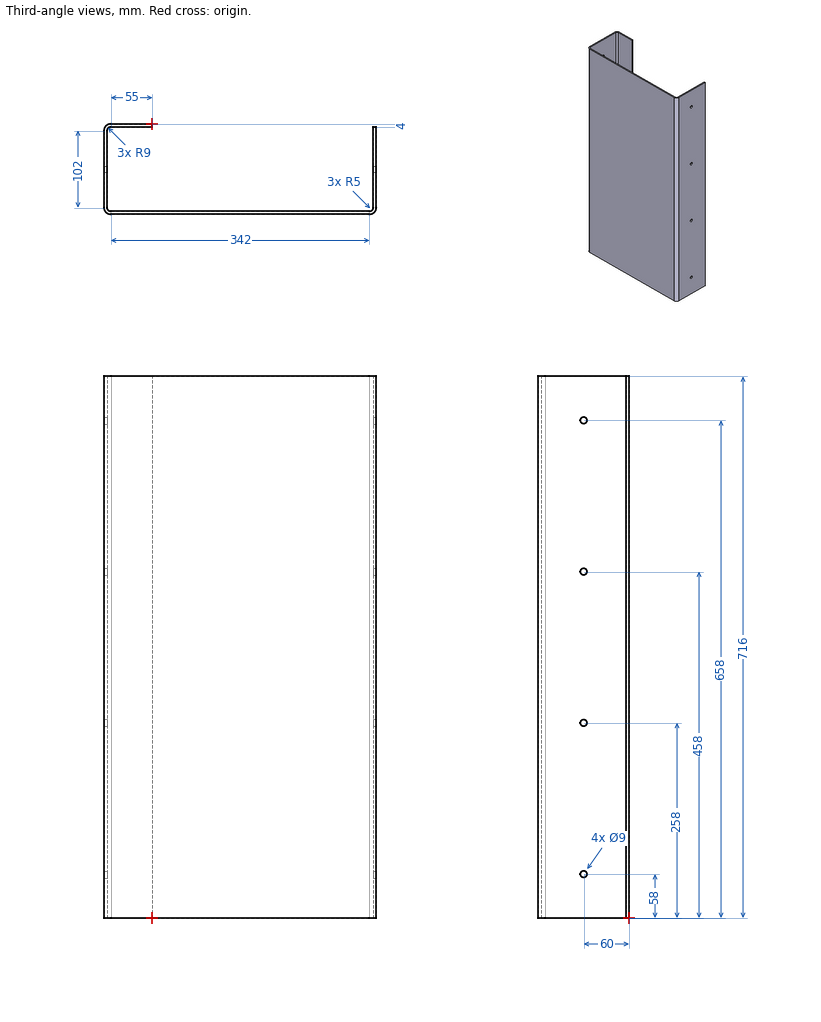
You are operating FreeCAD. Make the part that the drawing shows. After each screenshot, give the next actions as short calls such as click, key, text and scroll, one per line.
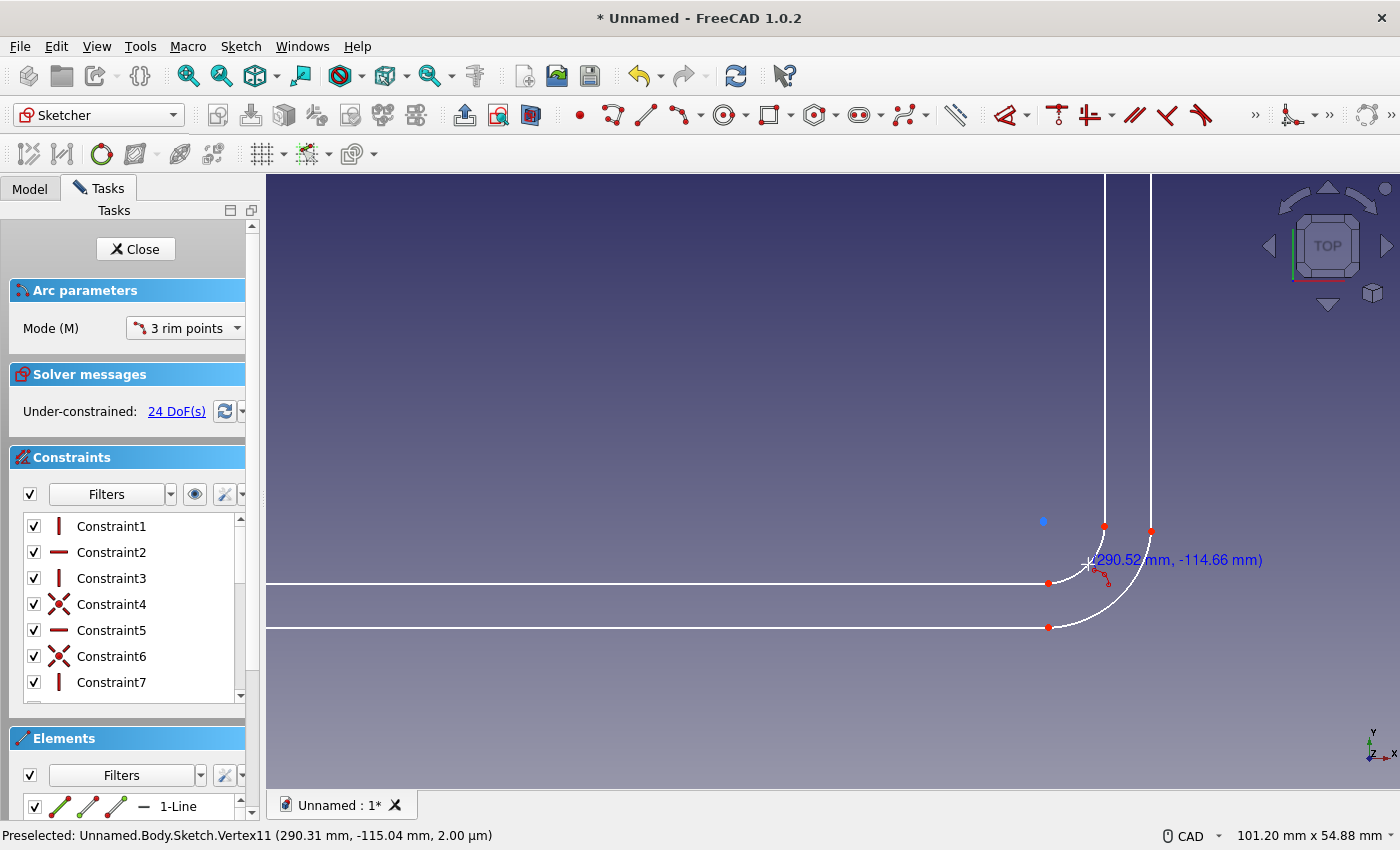
scroll(1088, 586, down, 9)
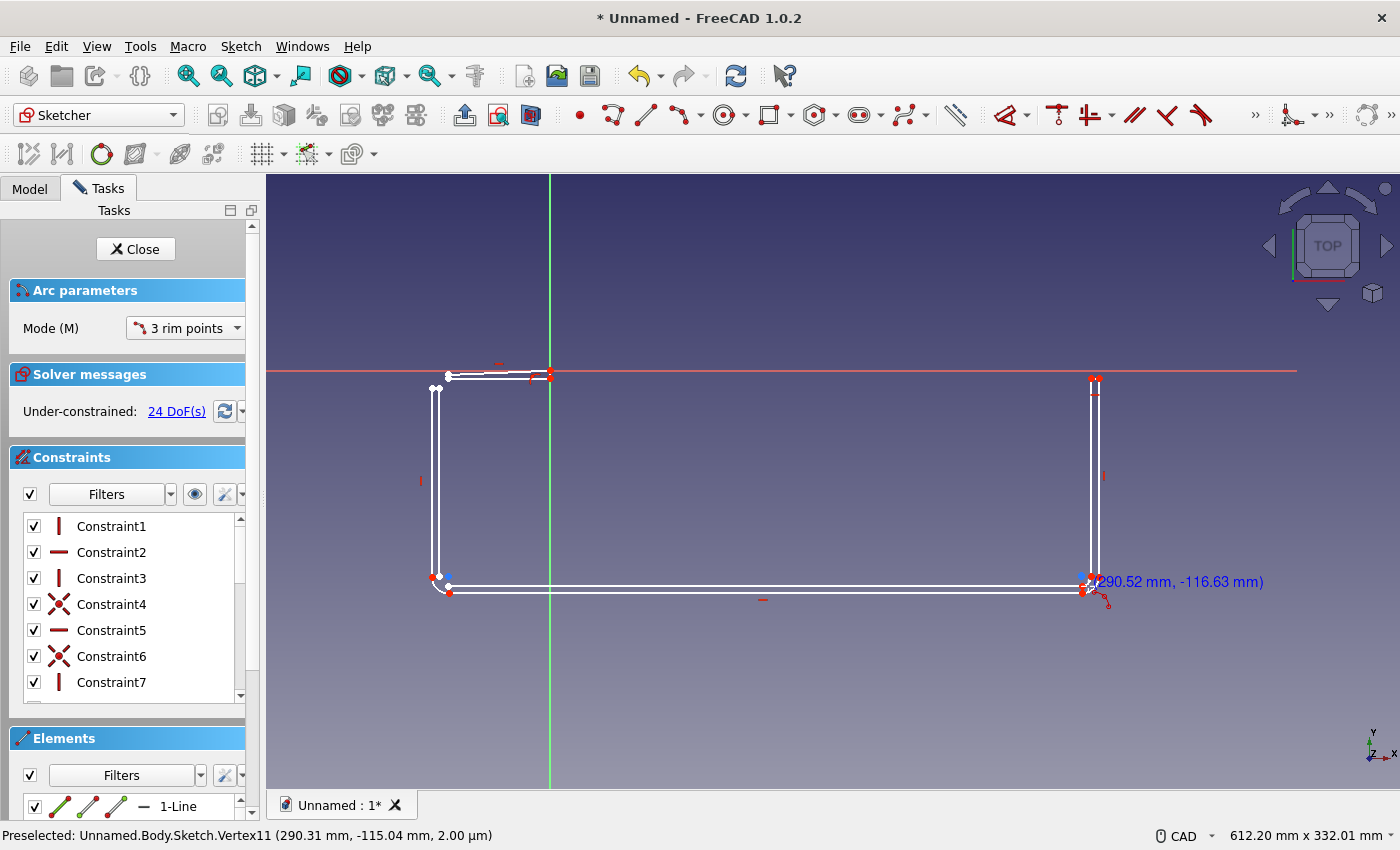
scroll(449, 586, up, 4)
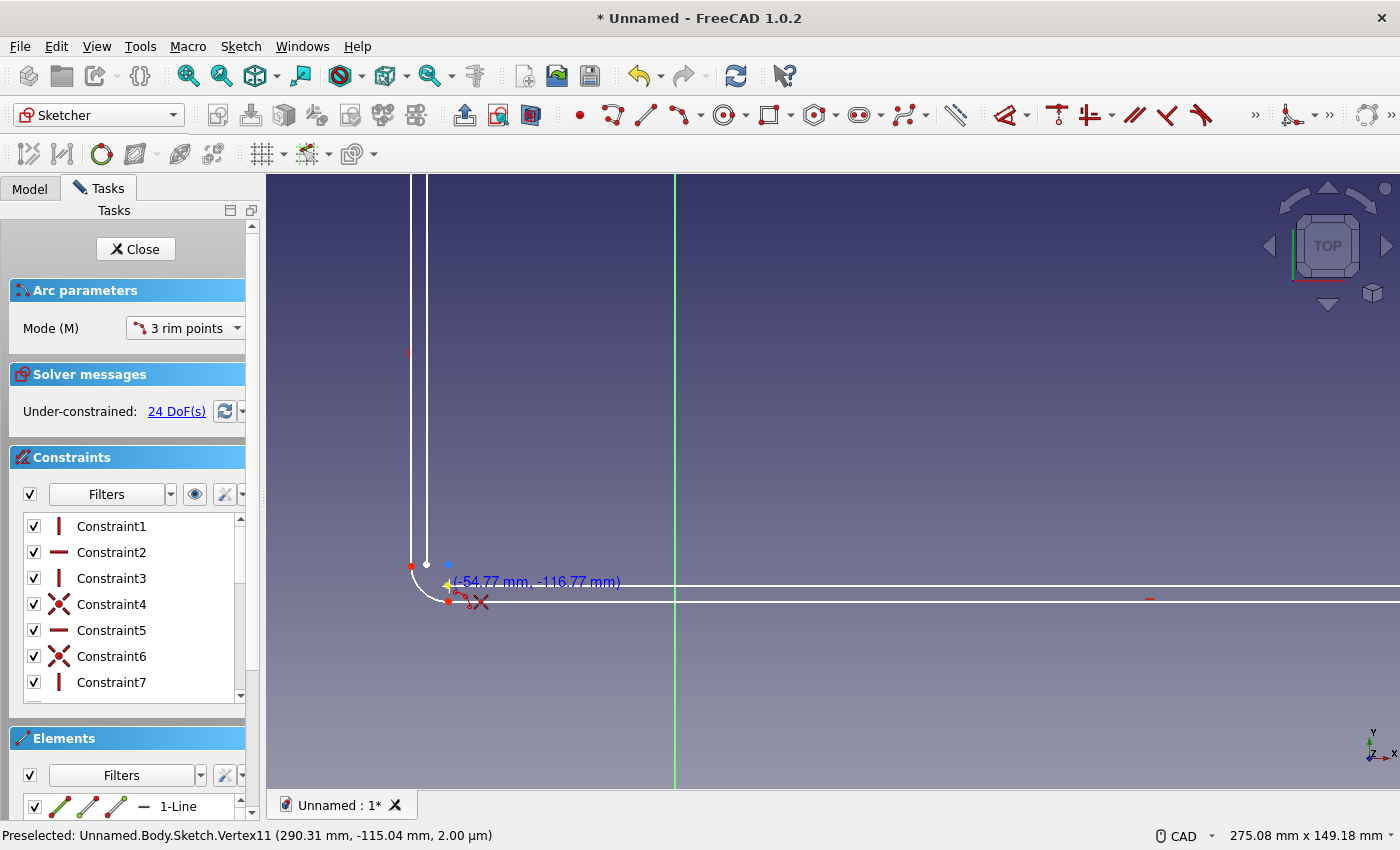
click(448, 586)
click(427, 565)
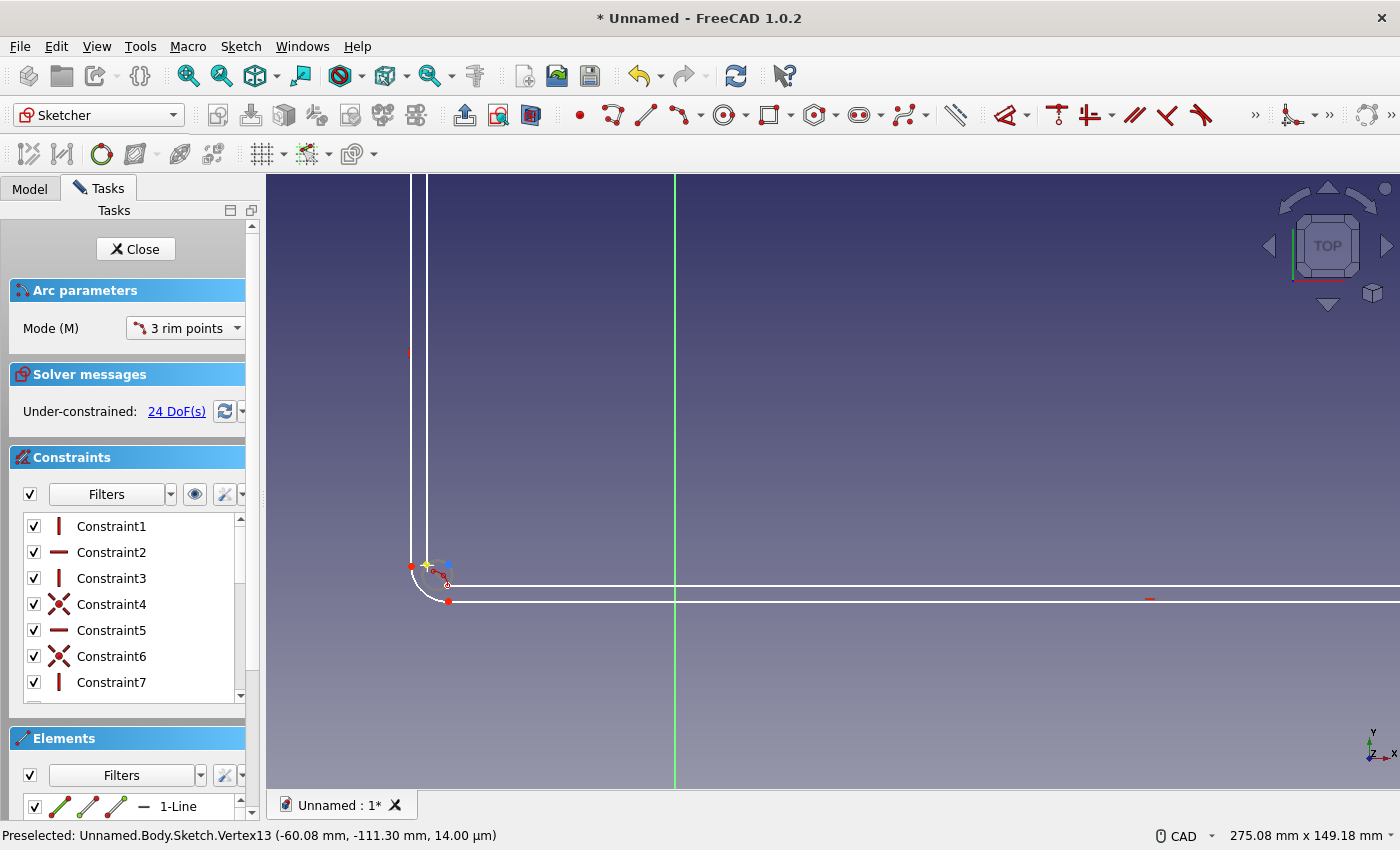
scroll(433, 578, up, 5)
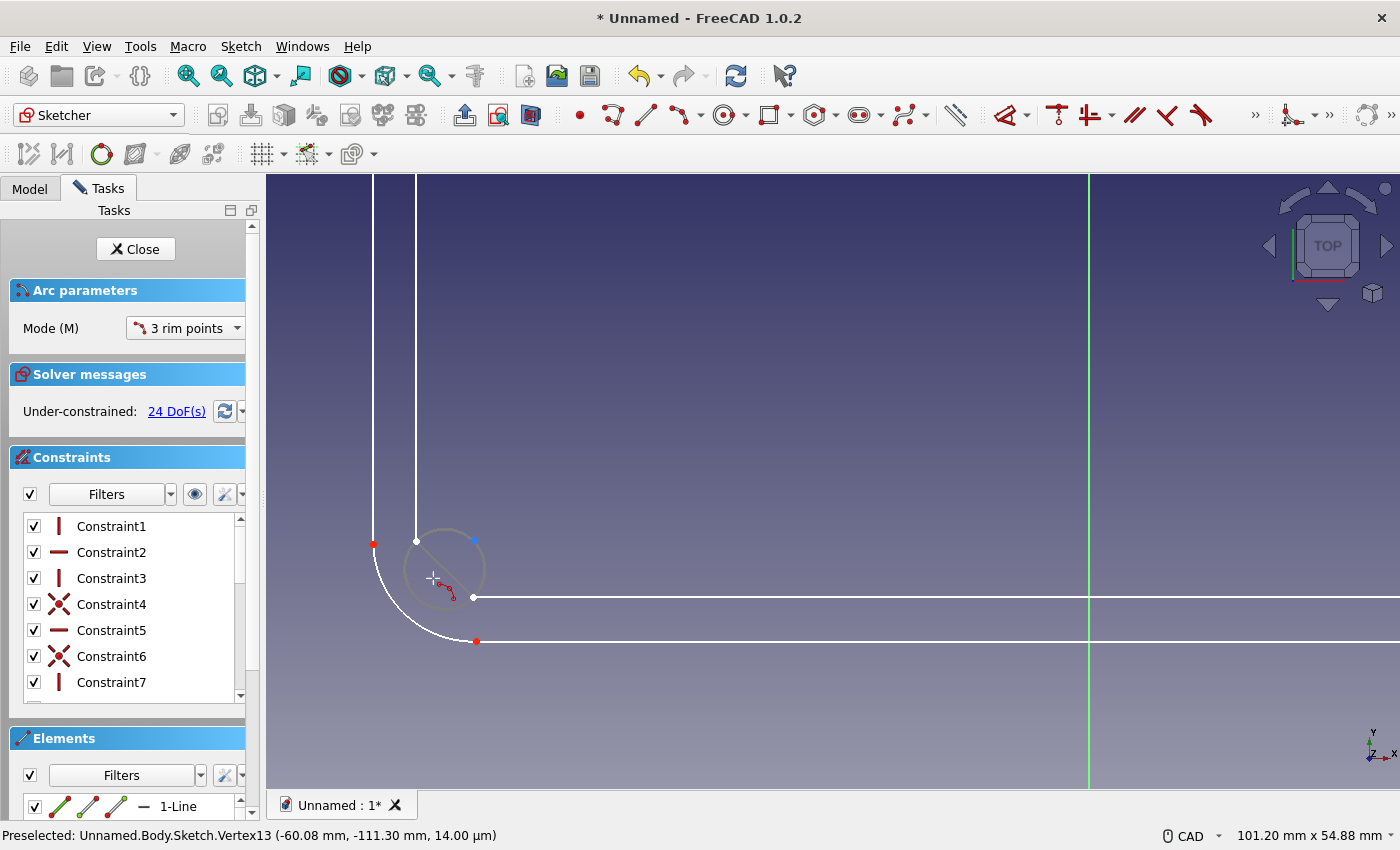
click(434, 577)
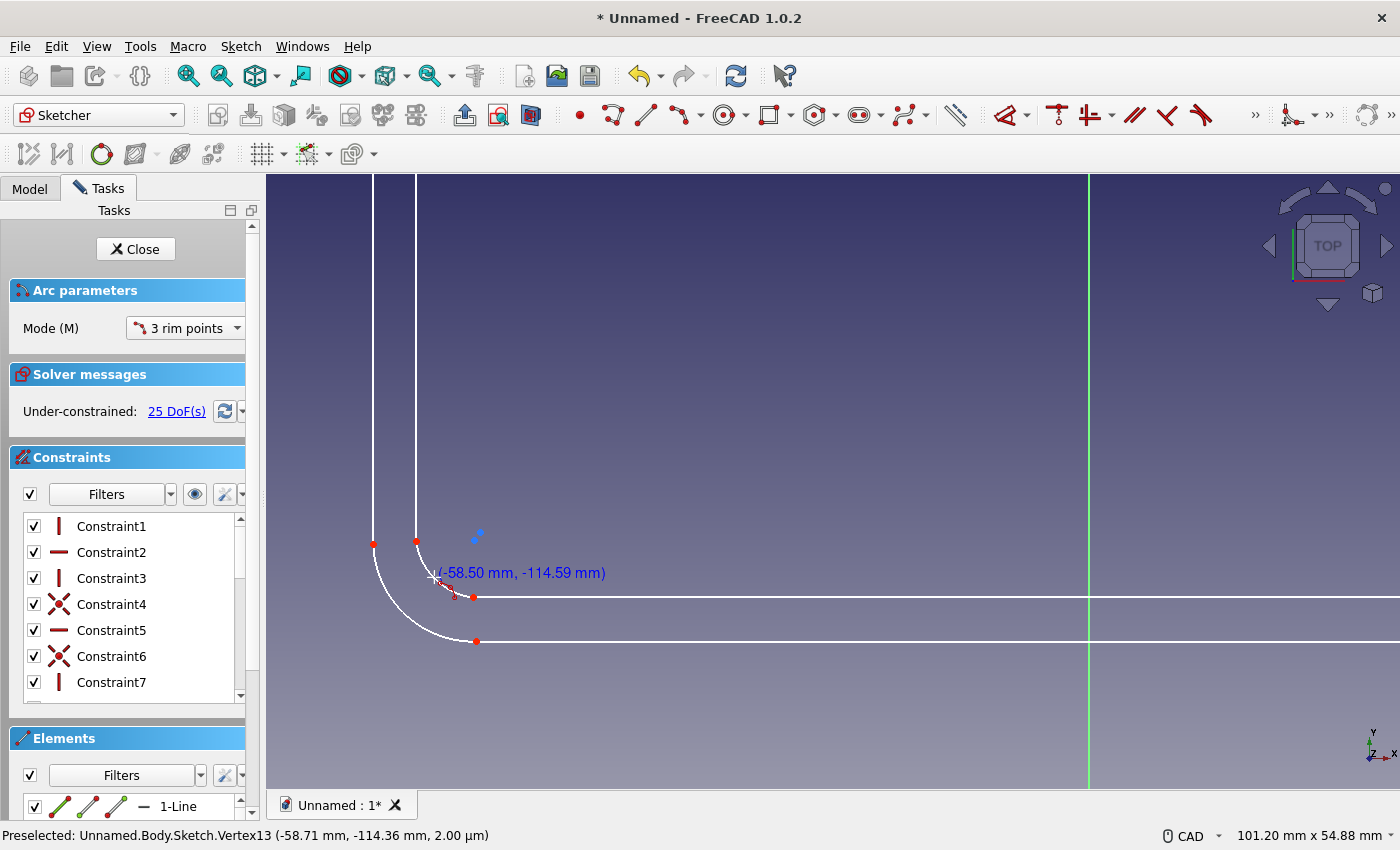
scroll(443, 584, down, 9)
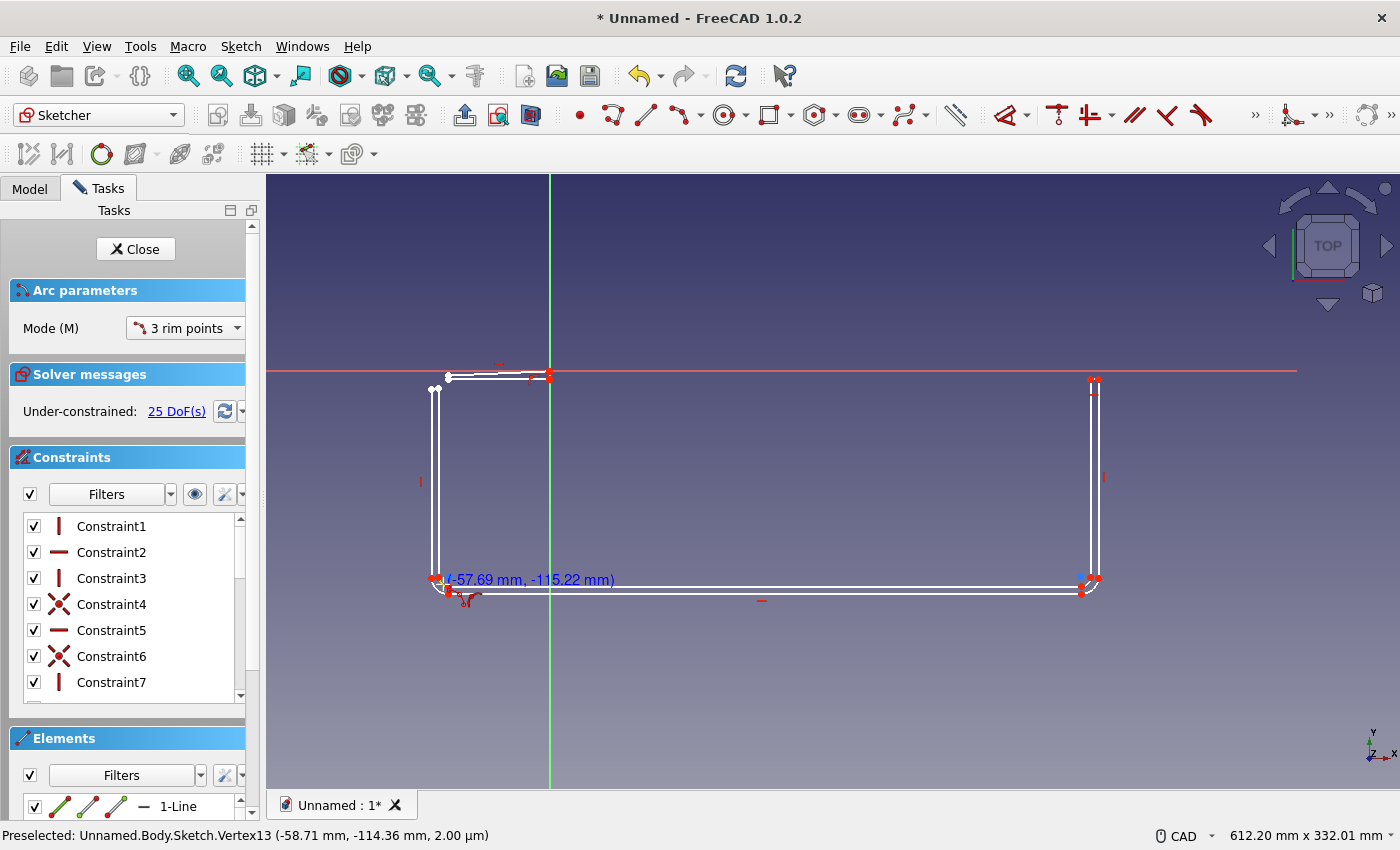
scroll(439, 388, up, 4)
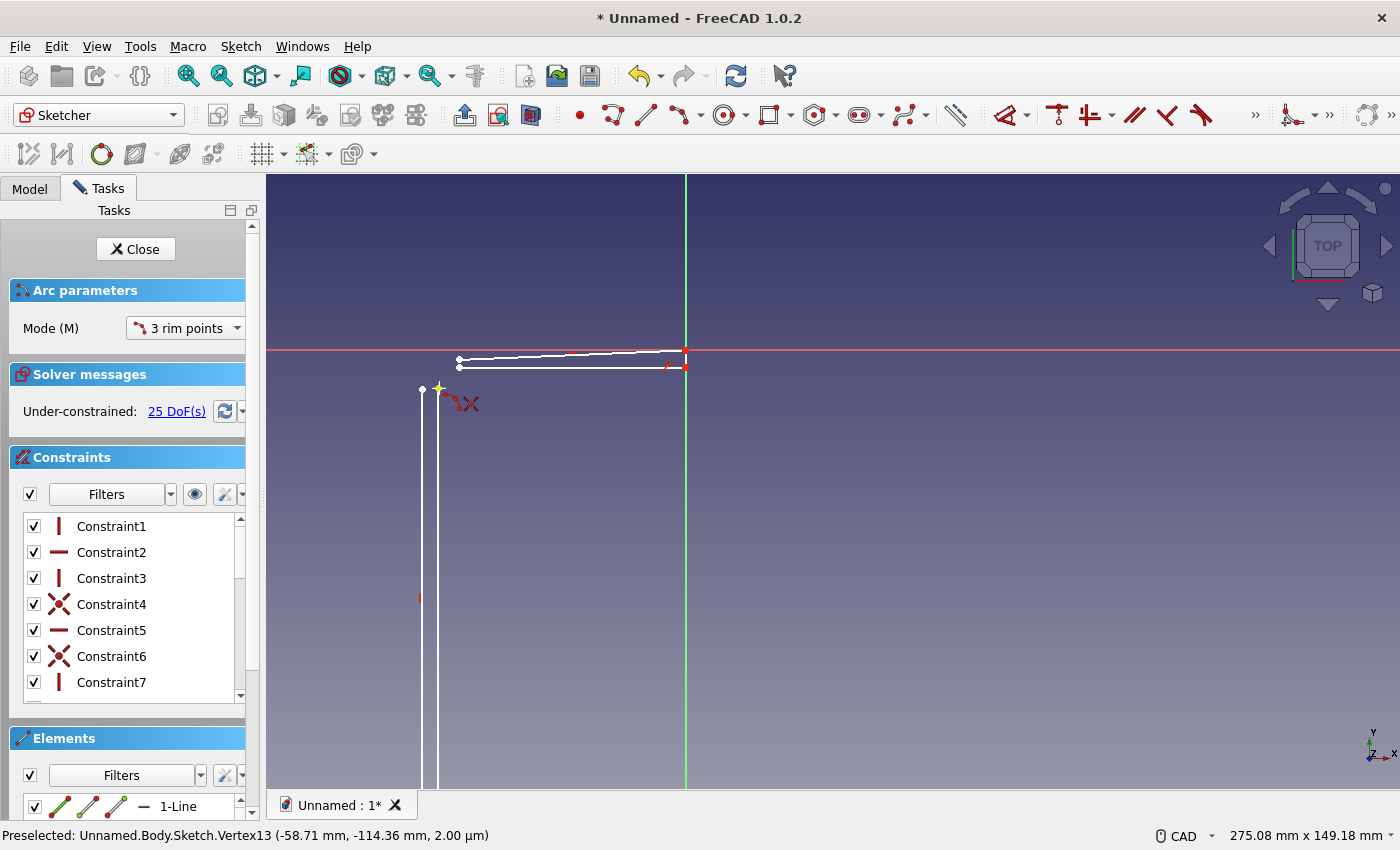
click(438, 389)
click(459, 368)